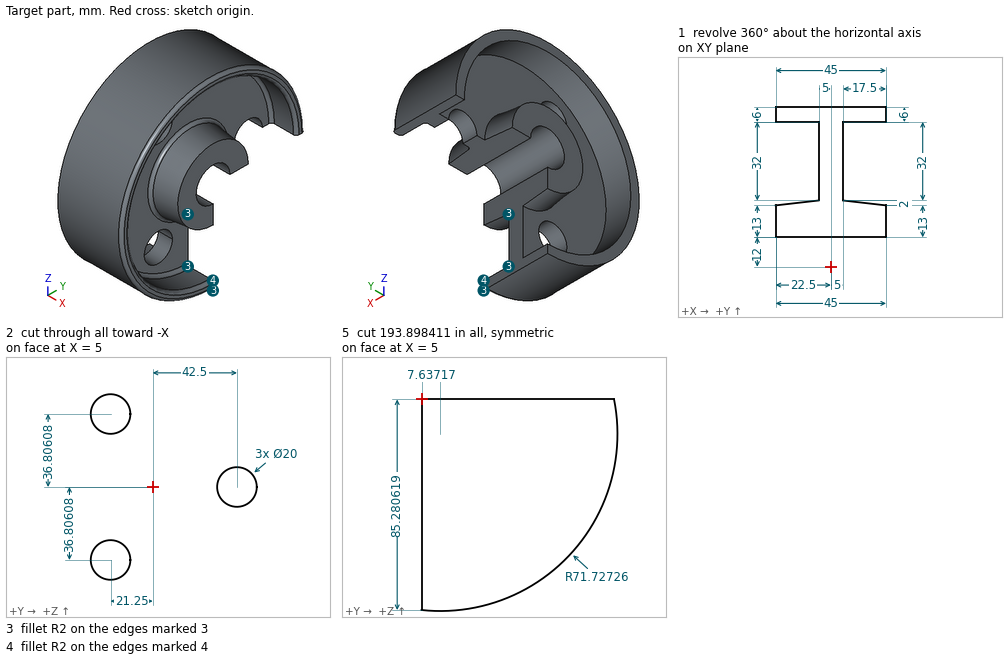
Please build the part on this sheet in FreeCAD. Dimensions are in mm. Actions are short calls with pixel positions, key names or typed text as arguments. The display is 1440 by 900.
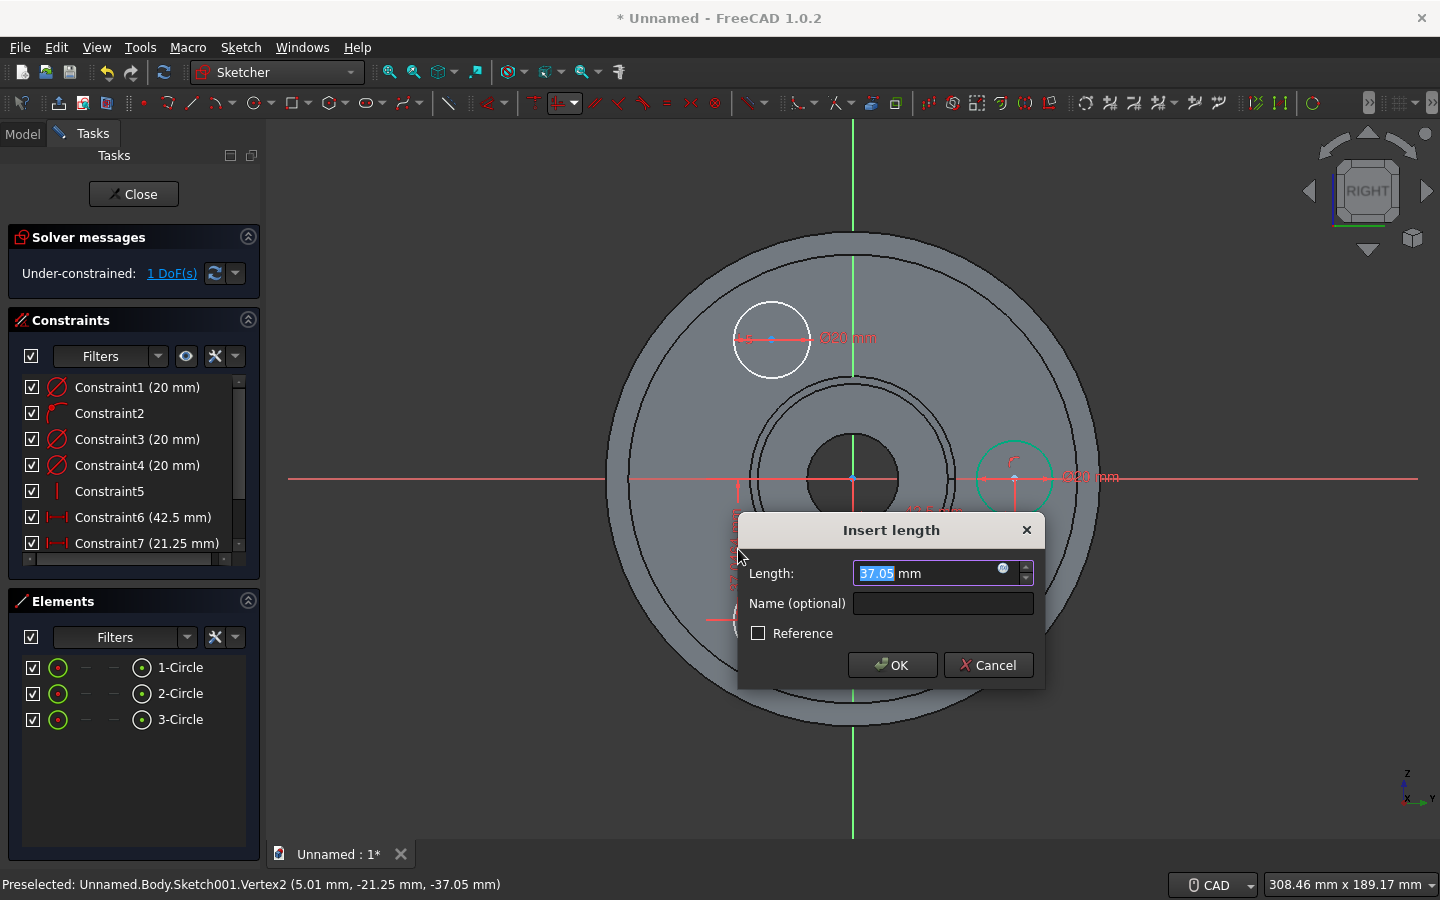
text(36.80608)
key(Return)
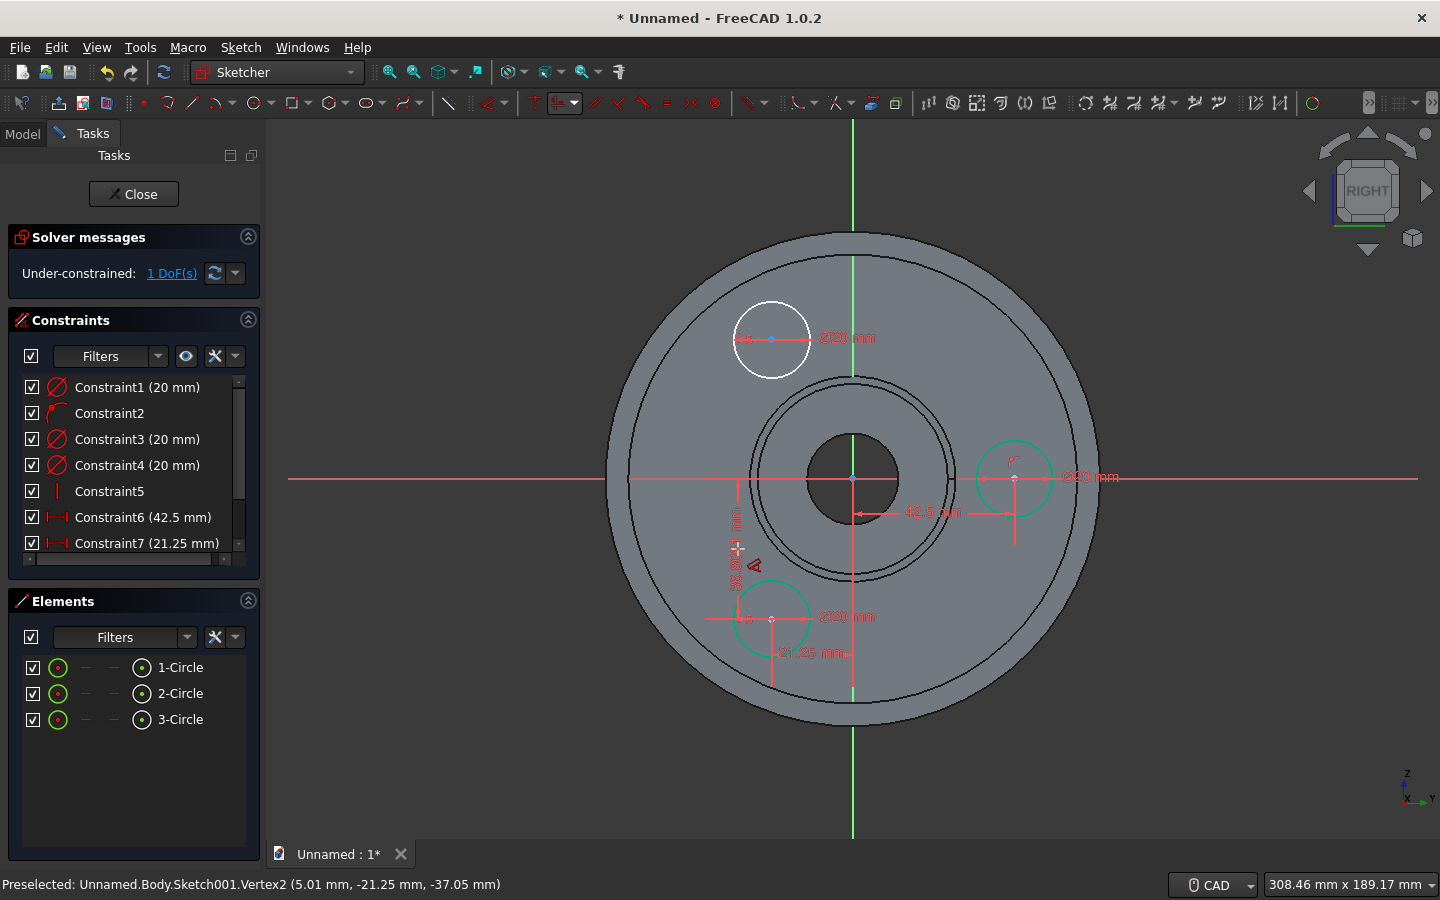
click(772, 340)
click(738, 409)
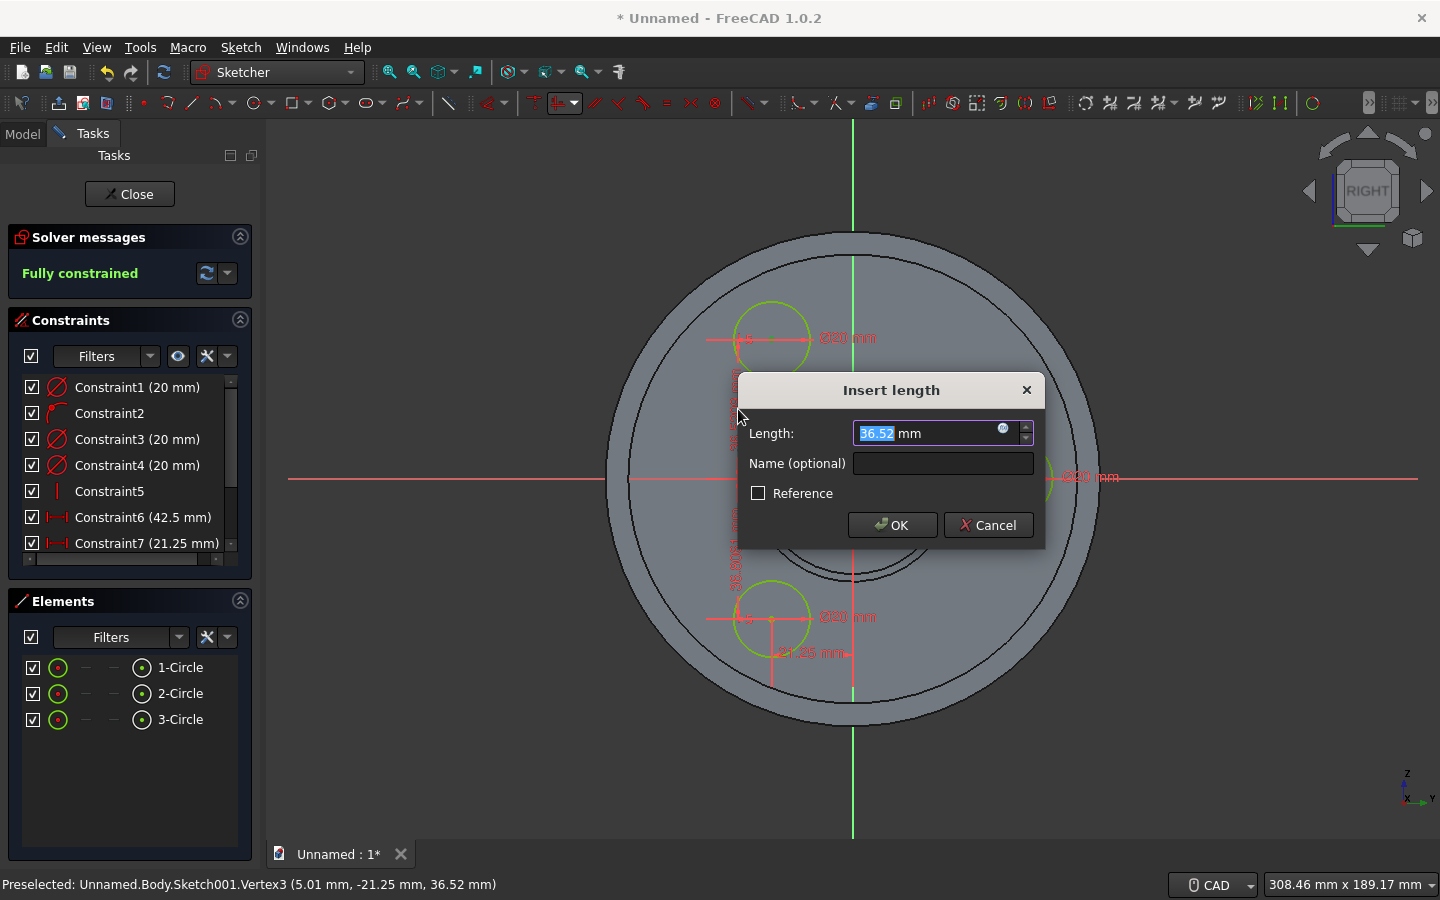
text(36.80608)
key(Return)
key(Escape)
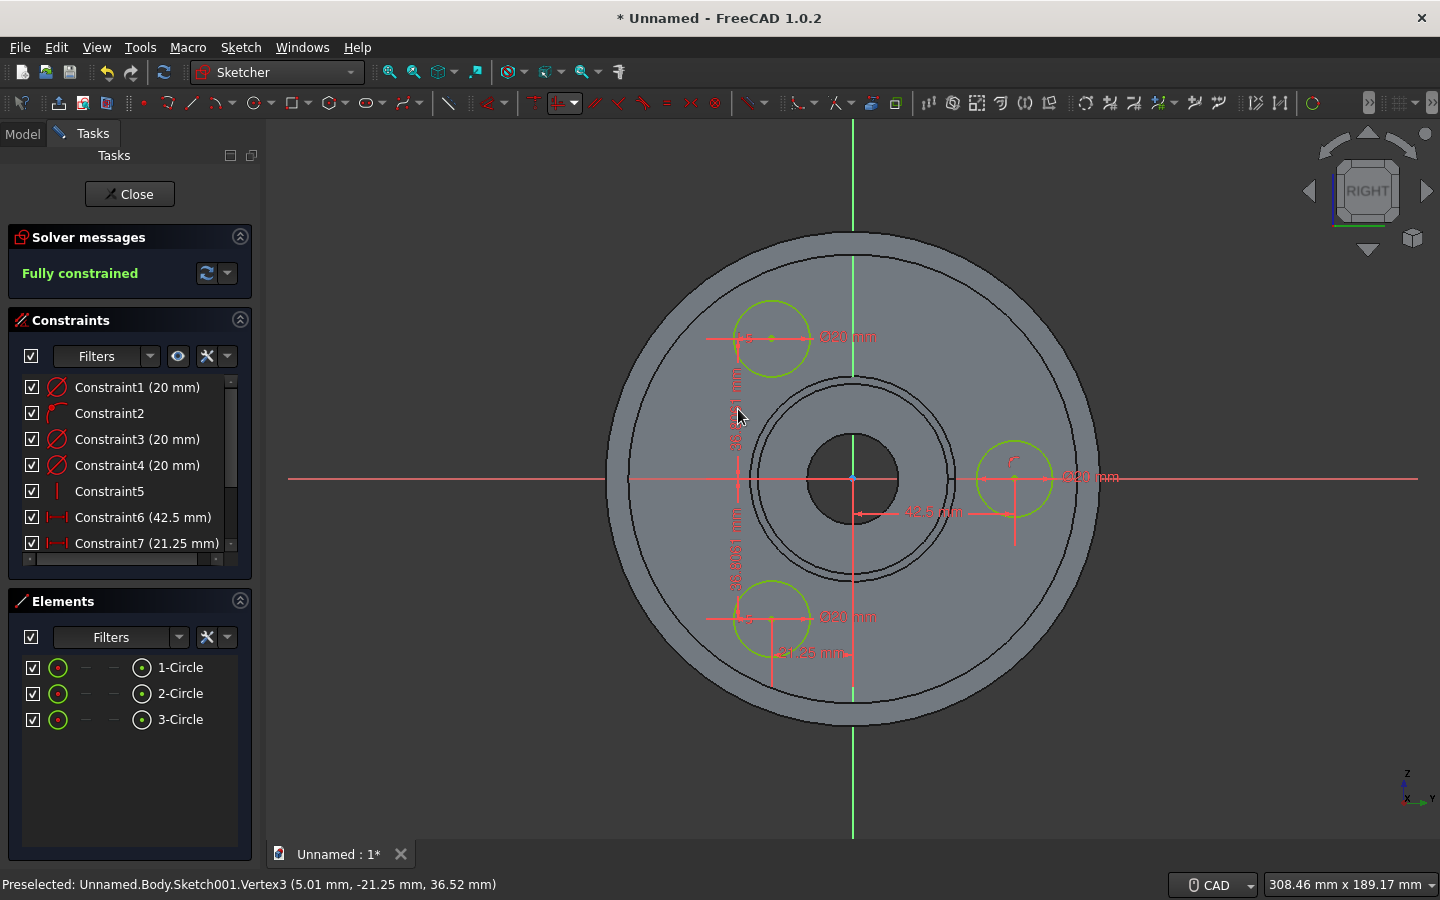
click(130, 194)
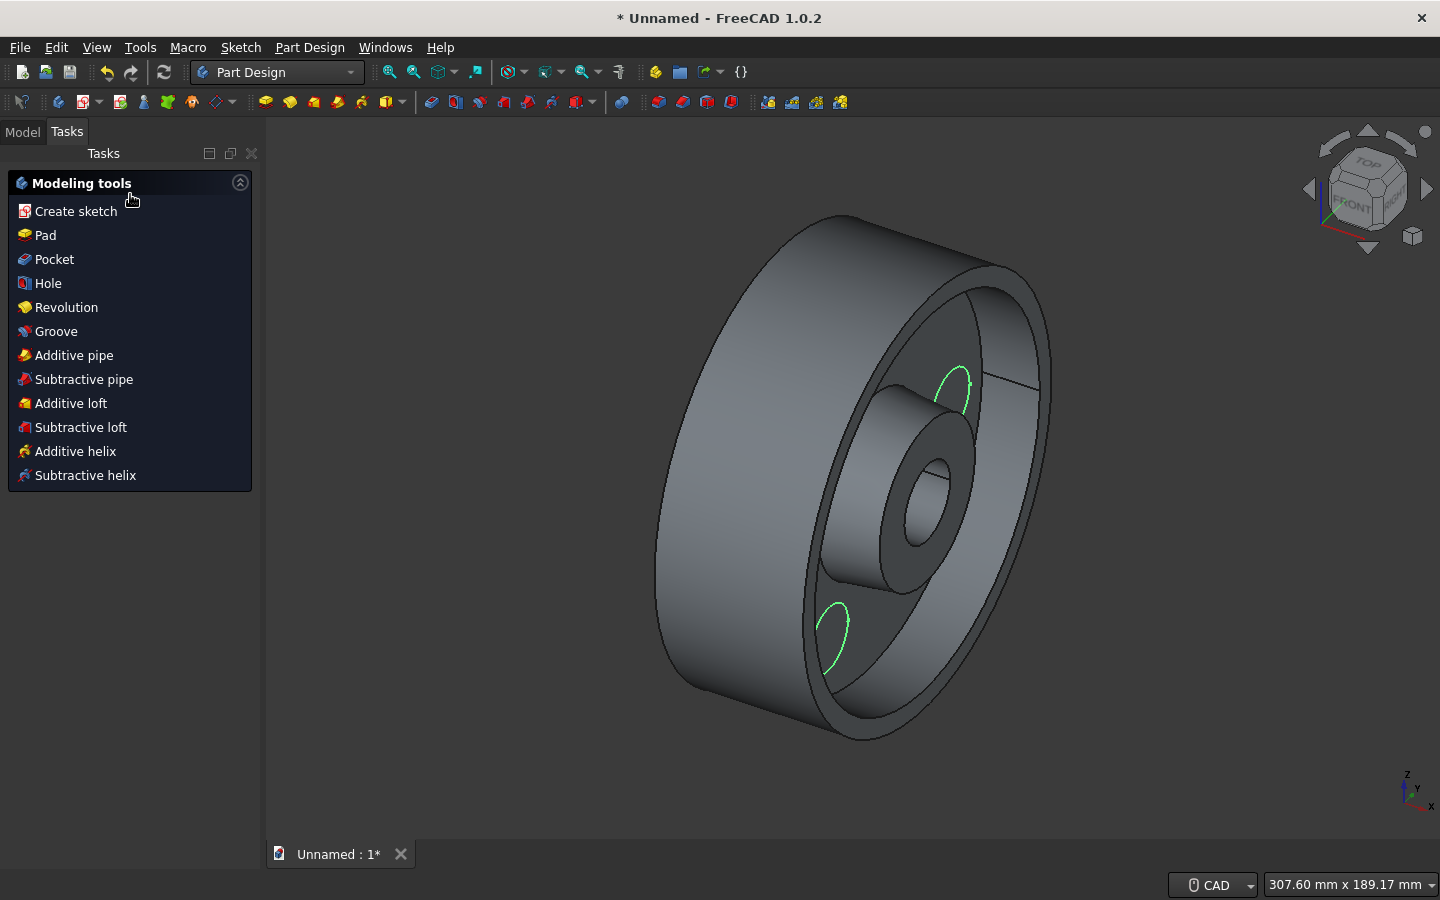
click(432, 102)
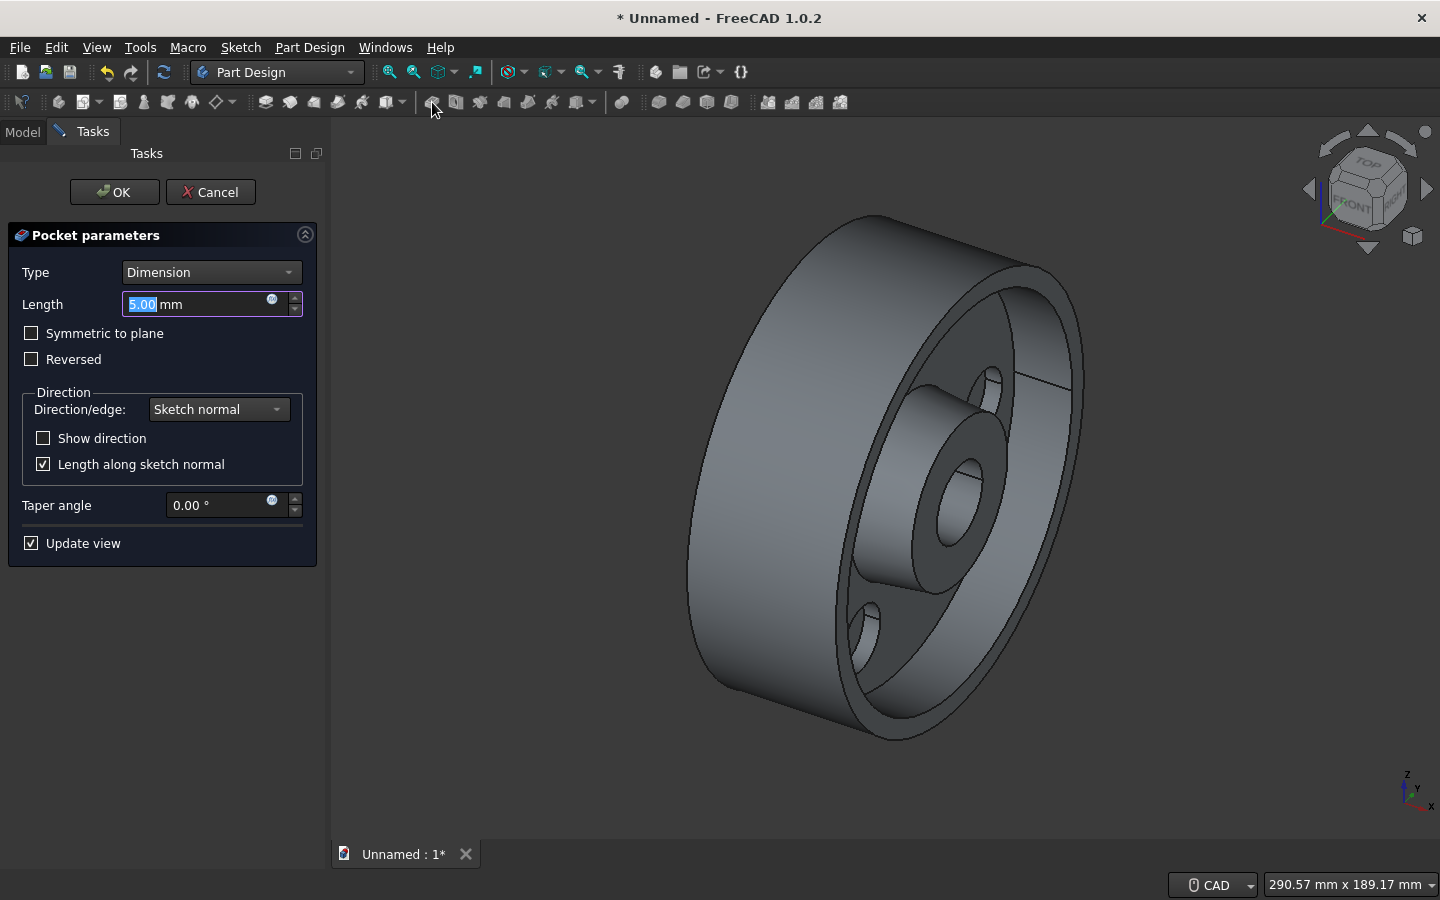
click(212, 272)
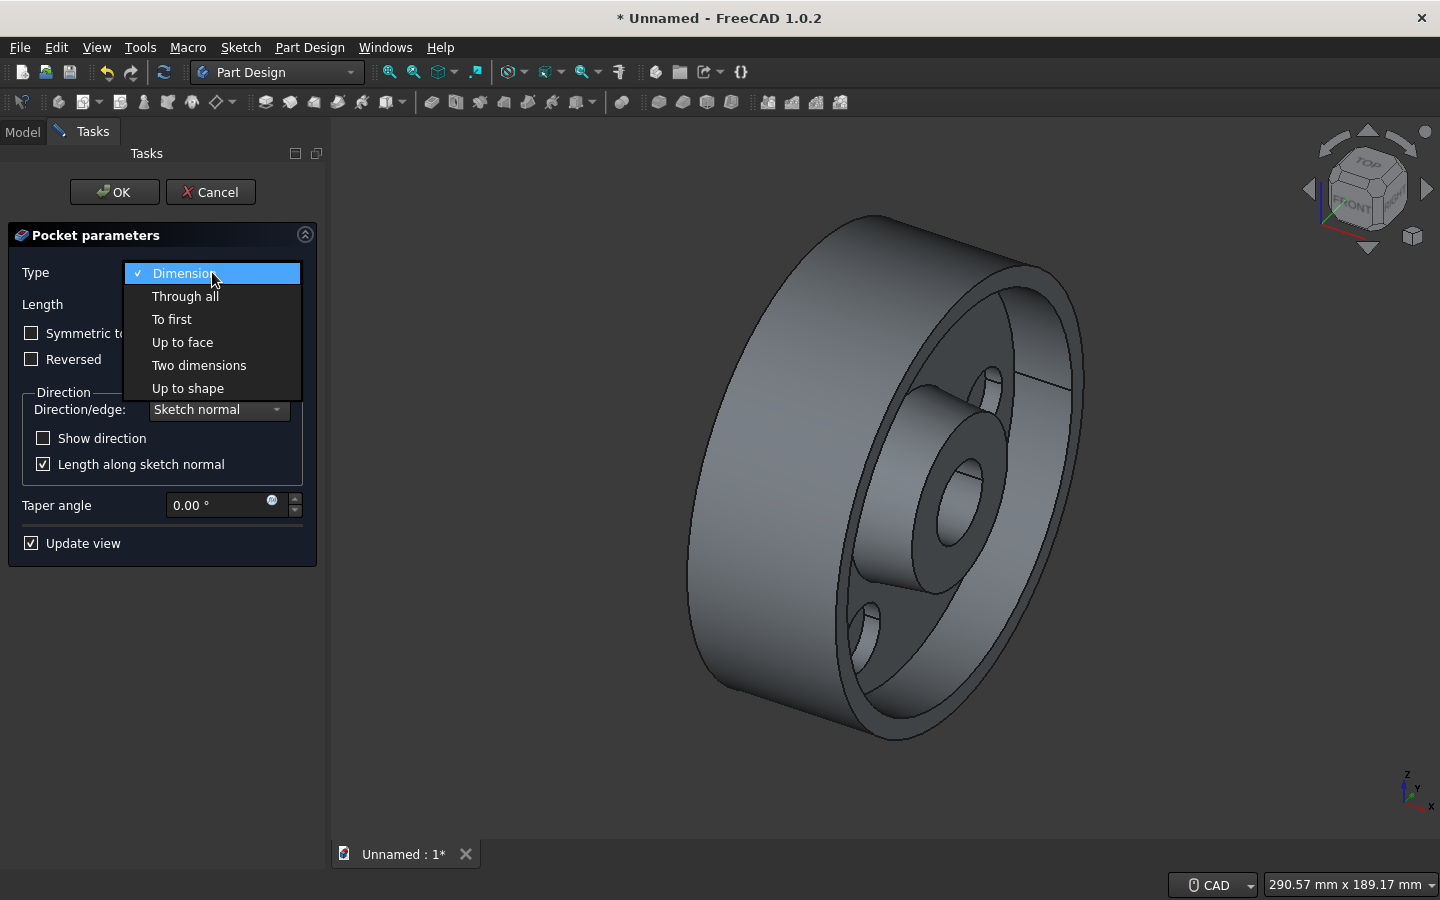
click(212, 296)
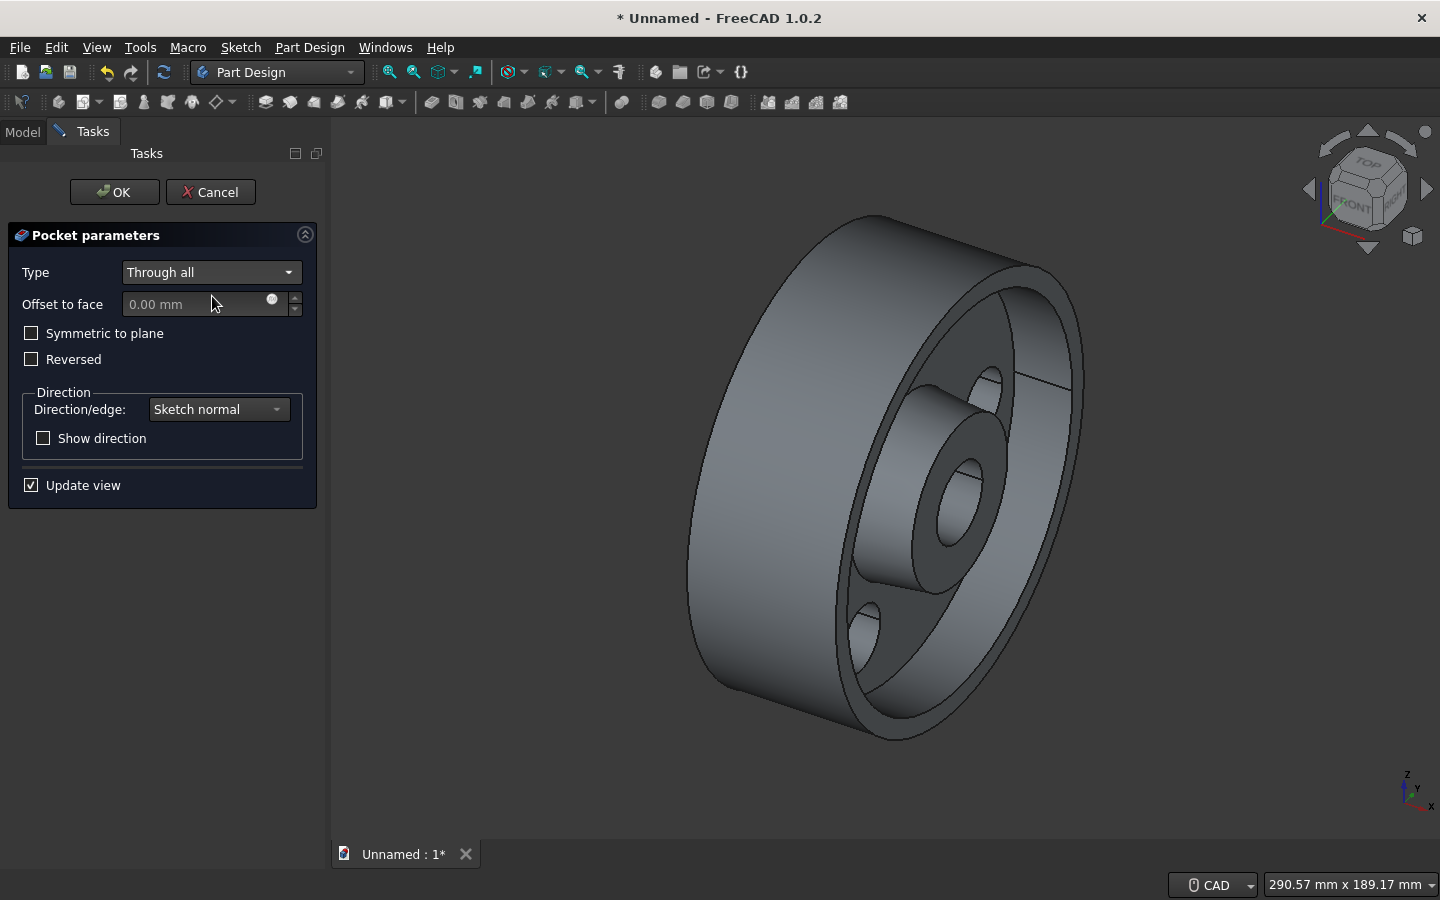
click(115, 192)